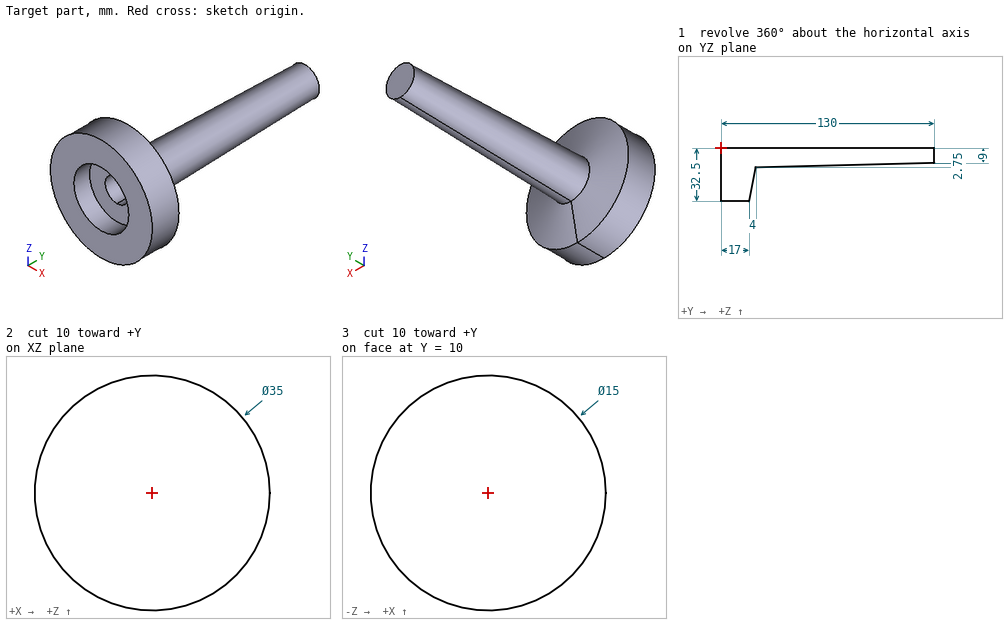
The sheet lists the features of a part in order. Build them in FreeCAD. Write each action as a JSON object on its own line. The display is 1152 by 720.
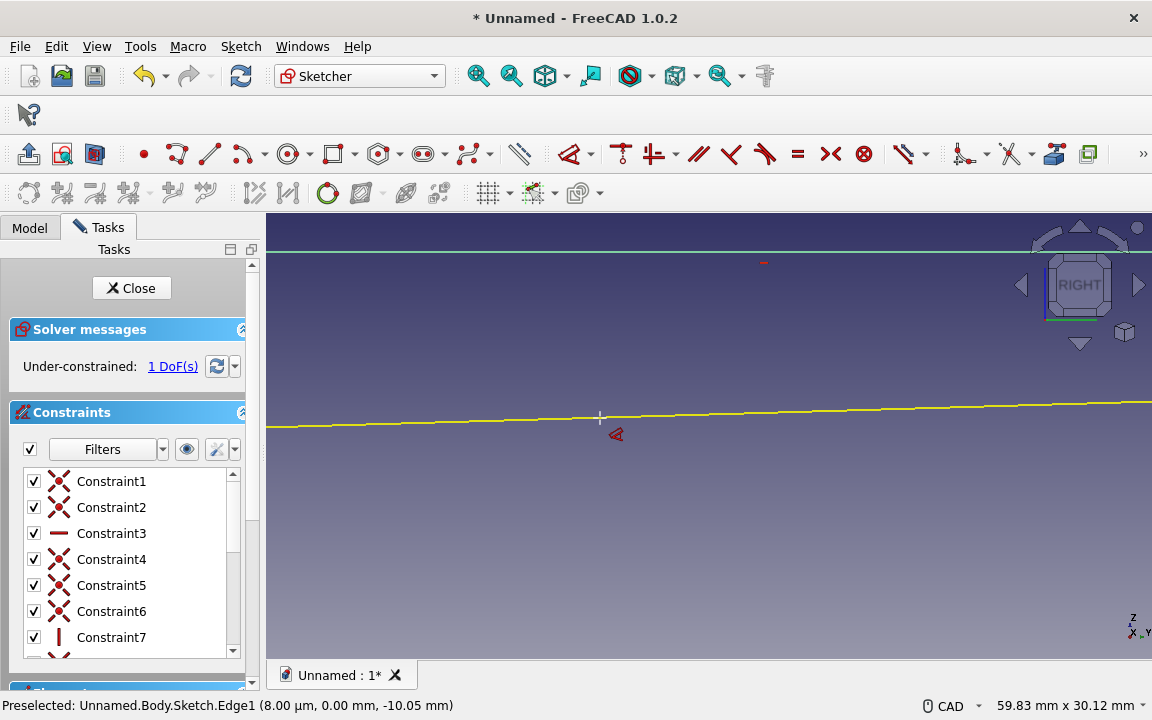
{"action": "left_click", "coordinate": [598, 418]}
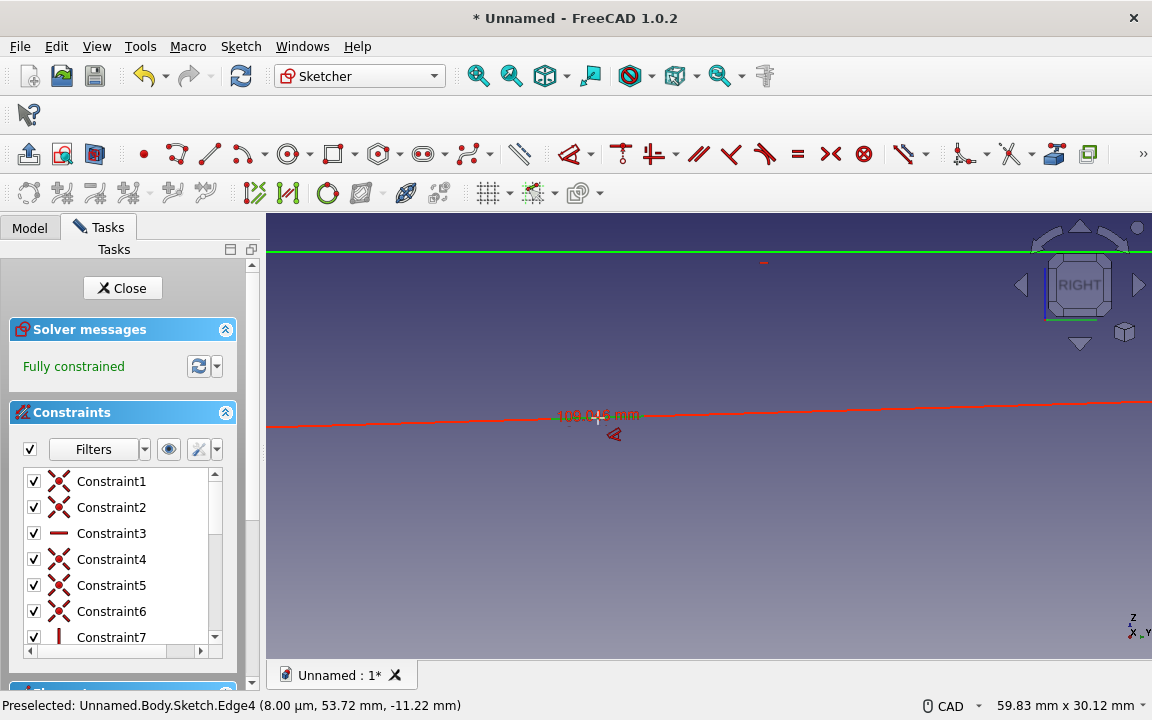
{"action": "key", "text": "Escape"}
{"action": "key", "text": "Escape"}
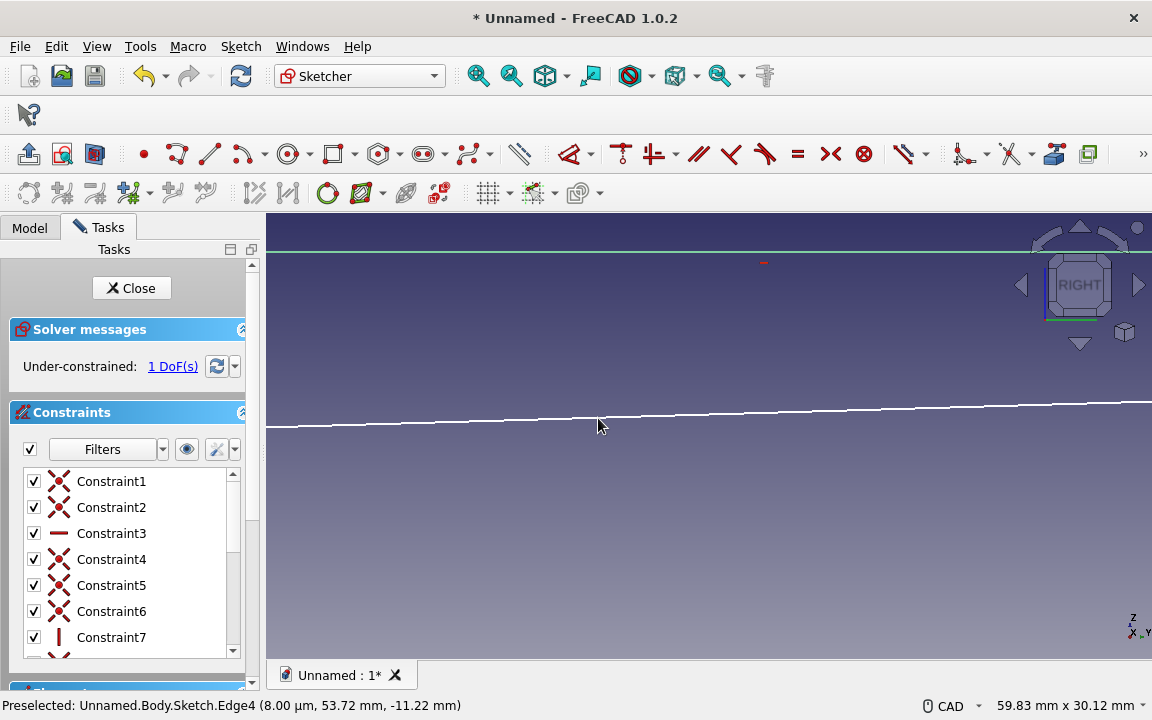
{"action": "left_click", "coordinate": [598, 418]}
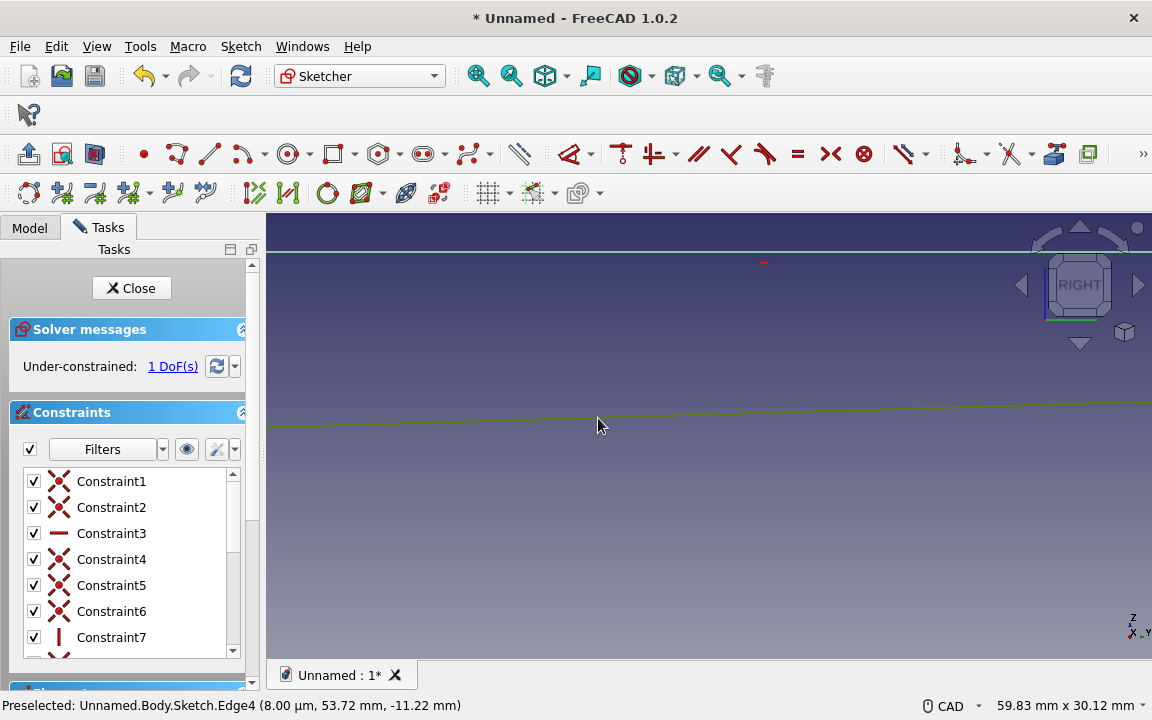
{"action": "left_click", "coordinate": [590, 154]}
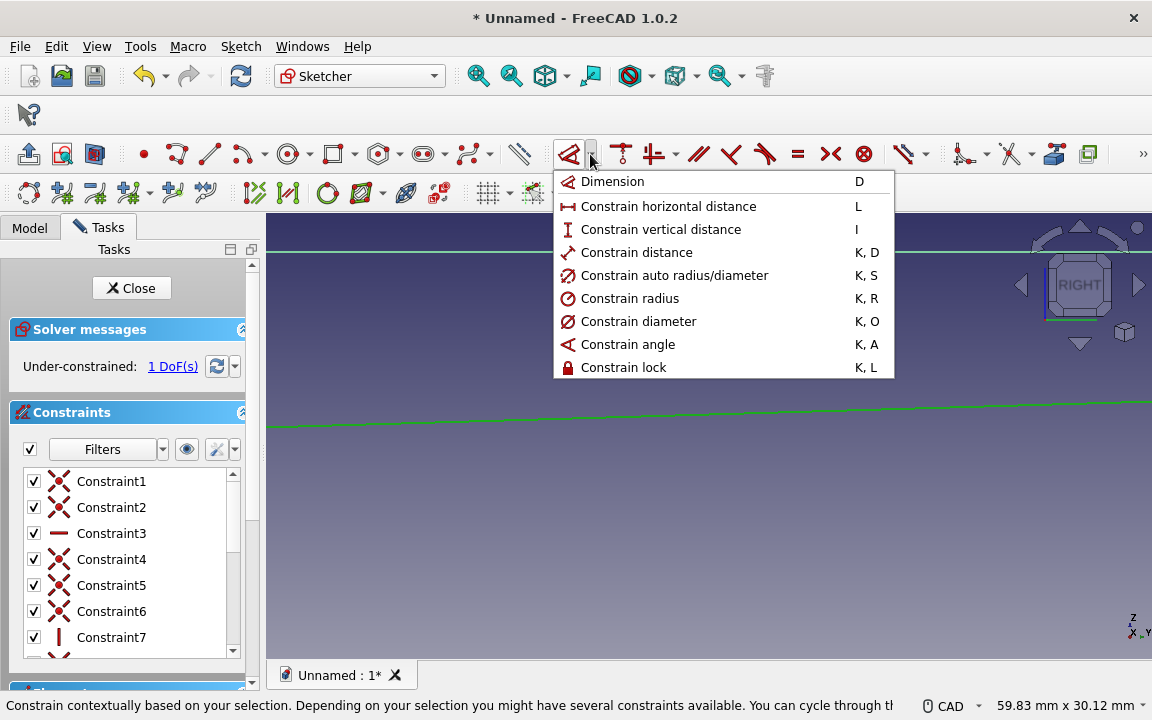
{"action": "left_click", "coordinate": [724, 230]}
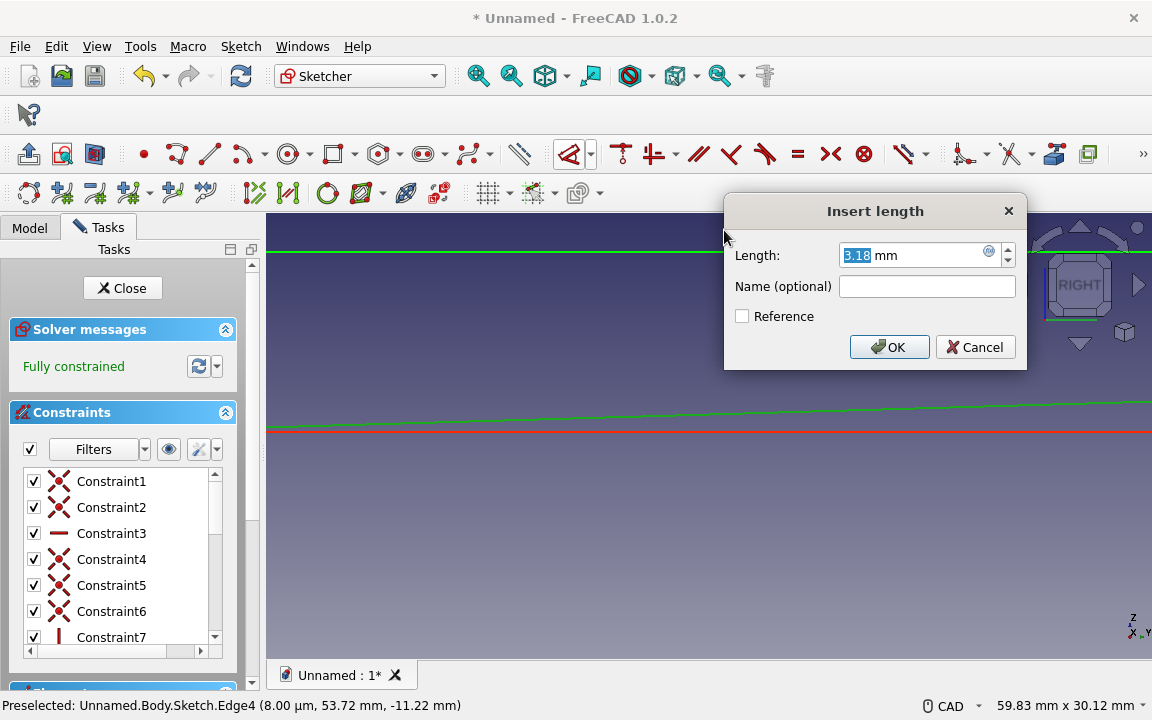
{"action": "type", "text": "2.75"}
{"action": "key", "text": "Return"}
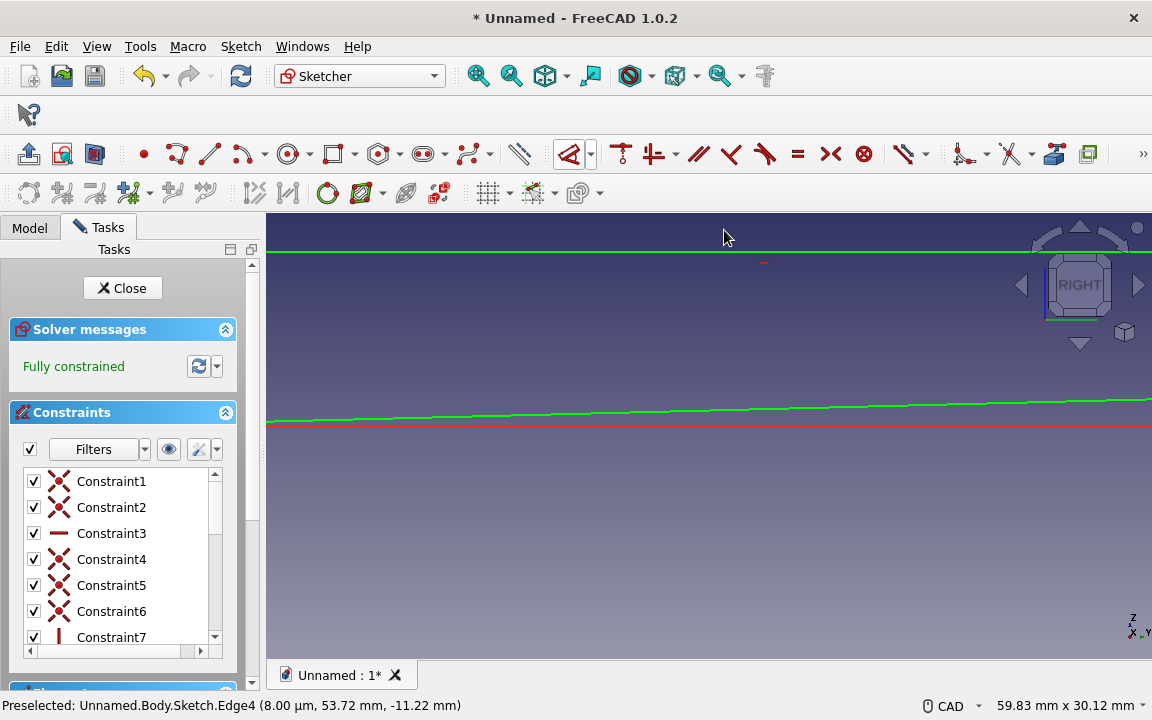
{"action": "left_click", "coordinate": [123, 288]}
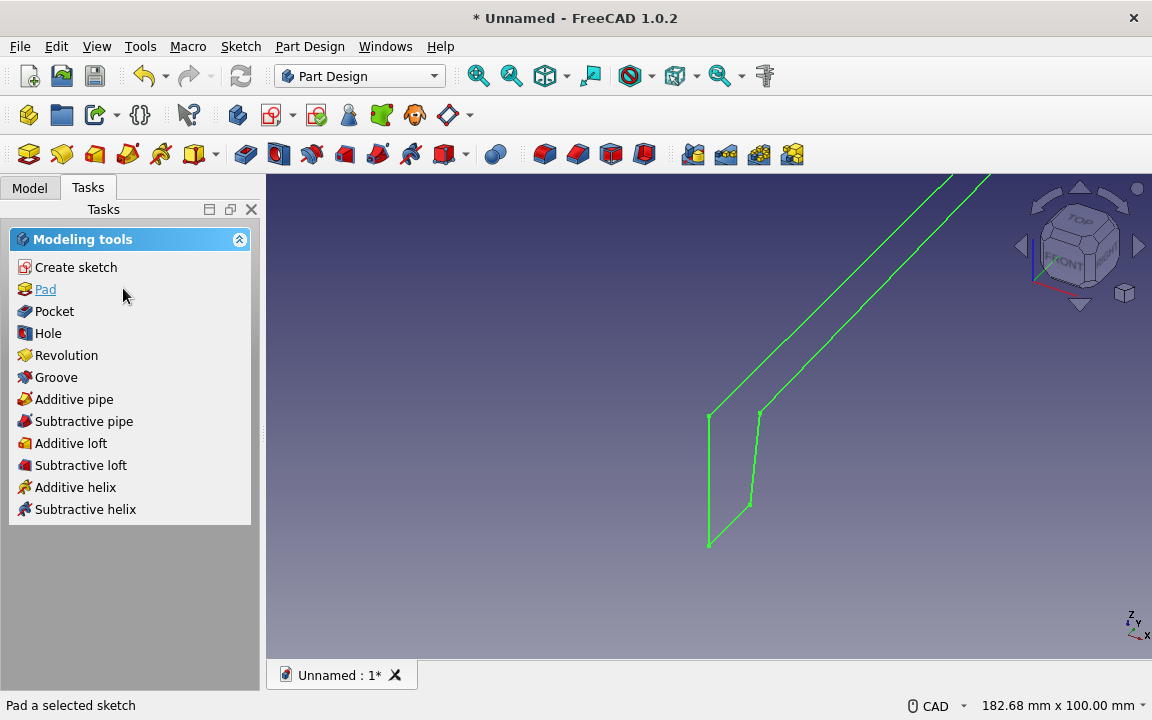
{"action": "left_click", "coordinate": [62, 154]}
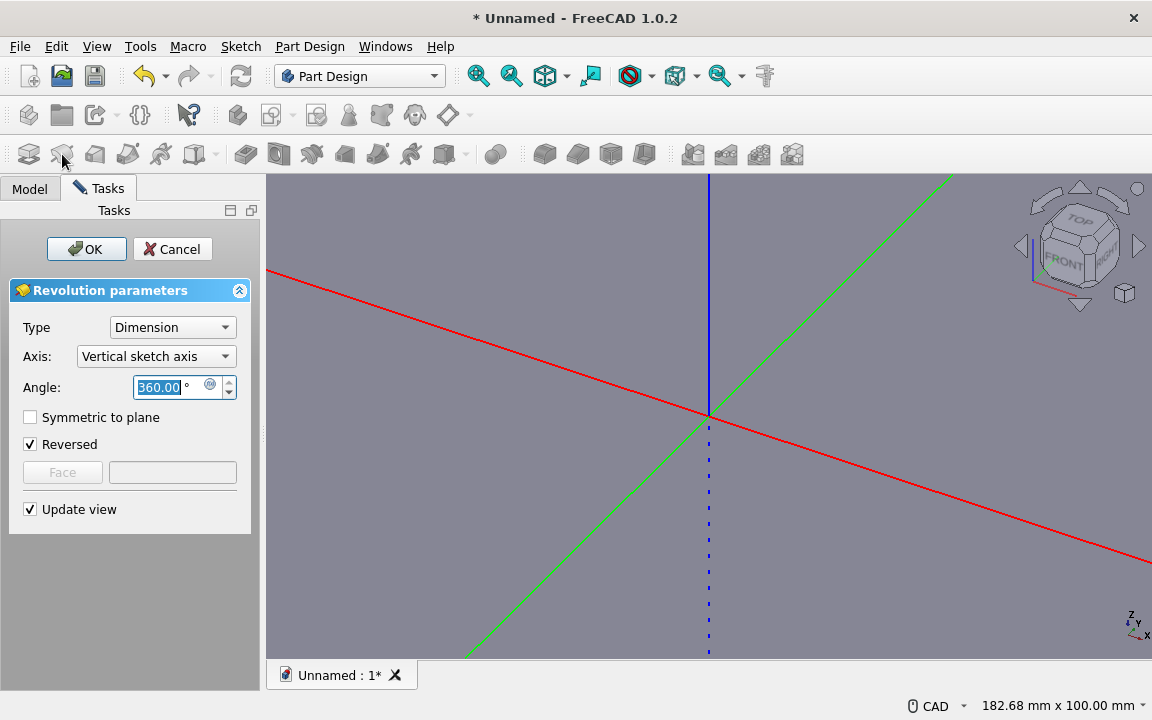
{"action": "left_click", "coordinate": [157, 356]}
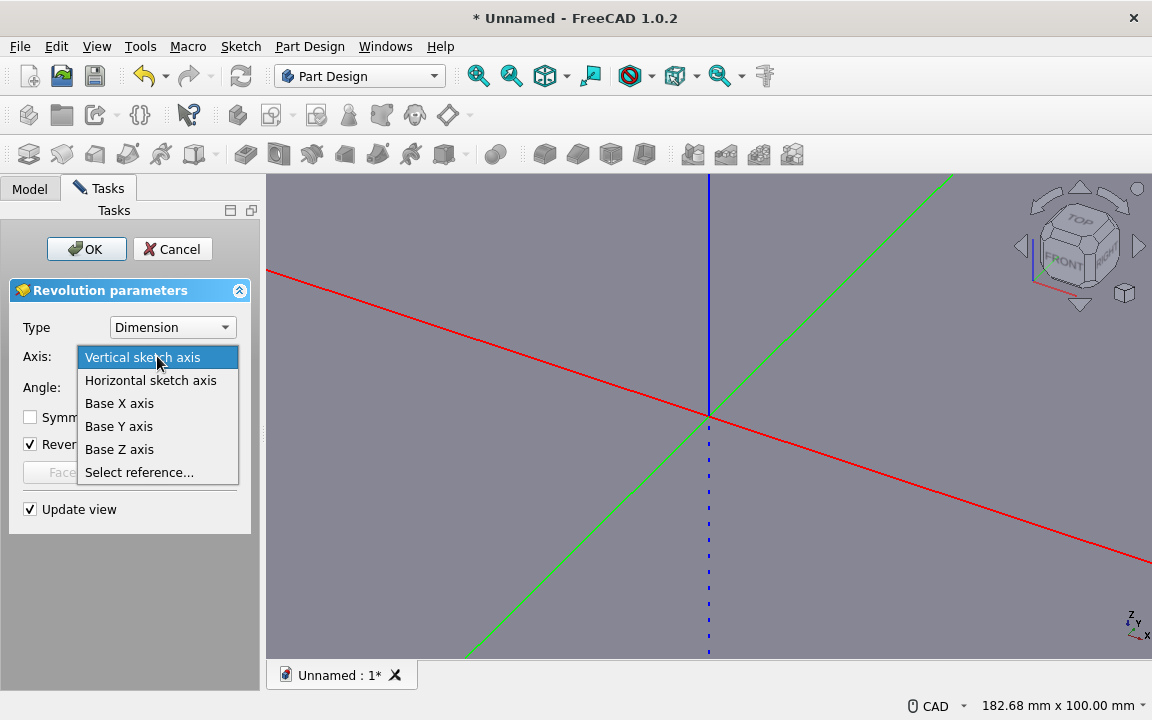
{"action": "left_click", "coordinate": [156, 380]}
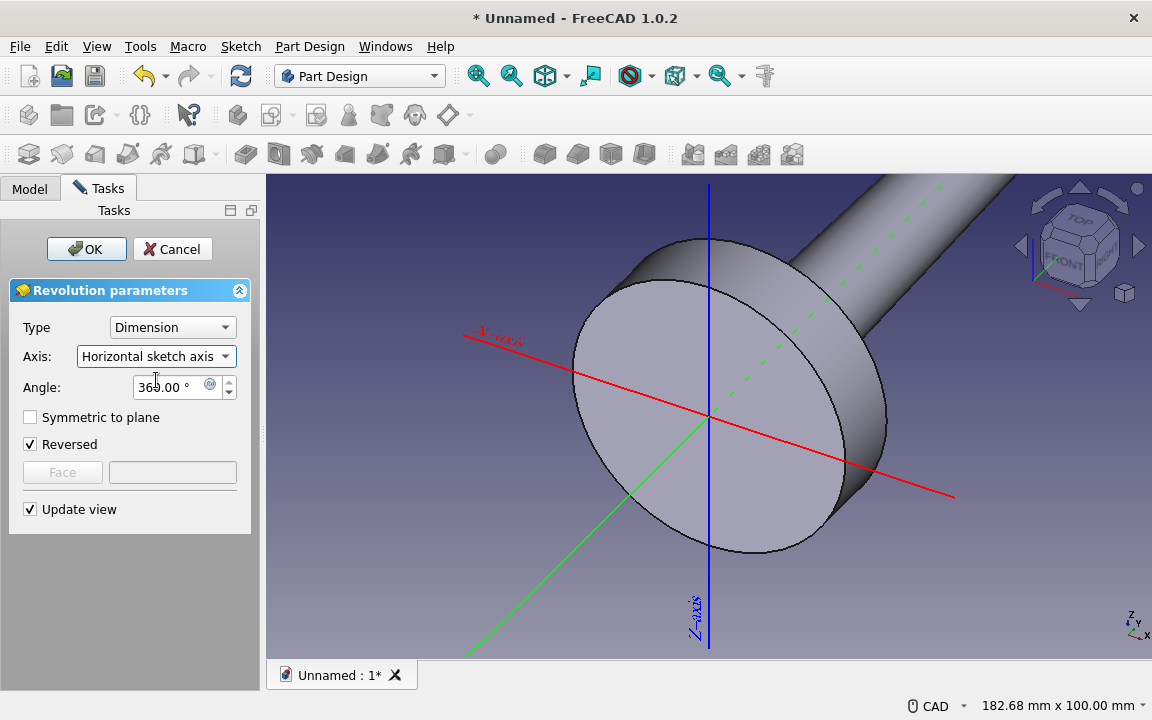
{"action": "left_click", "coordinate": [87, 249]}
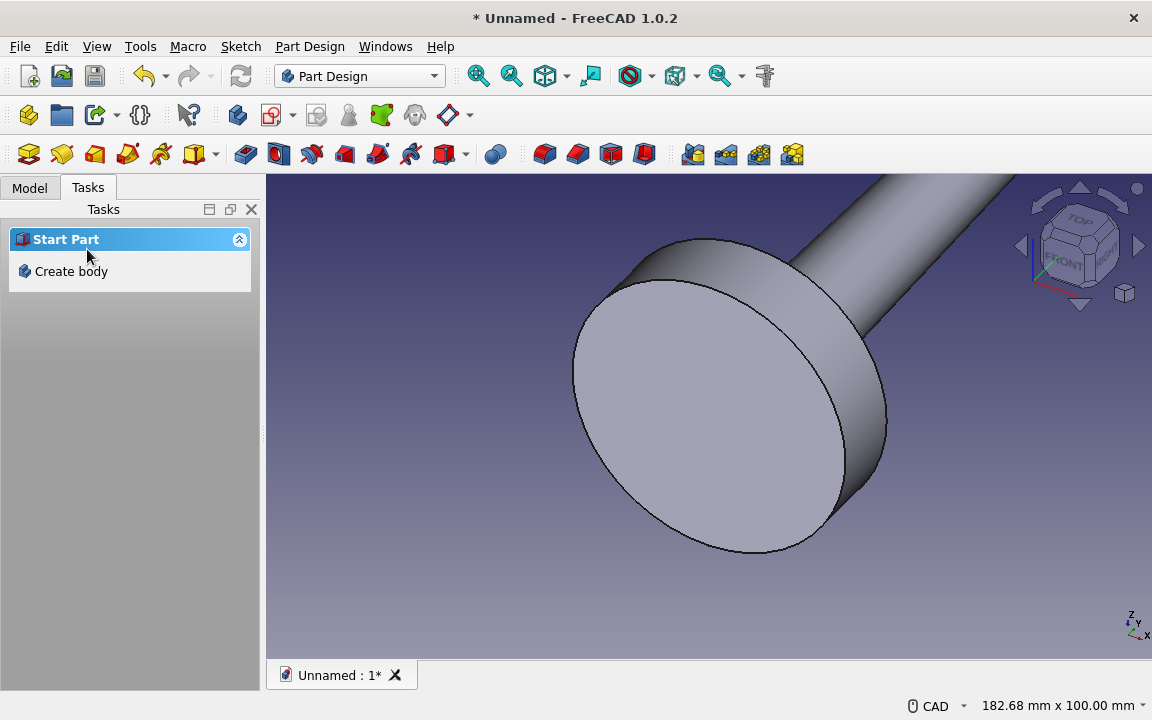
{"action": "left_click", "coordinate": [479, 76]}